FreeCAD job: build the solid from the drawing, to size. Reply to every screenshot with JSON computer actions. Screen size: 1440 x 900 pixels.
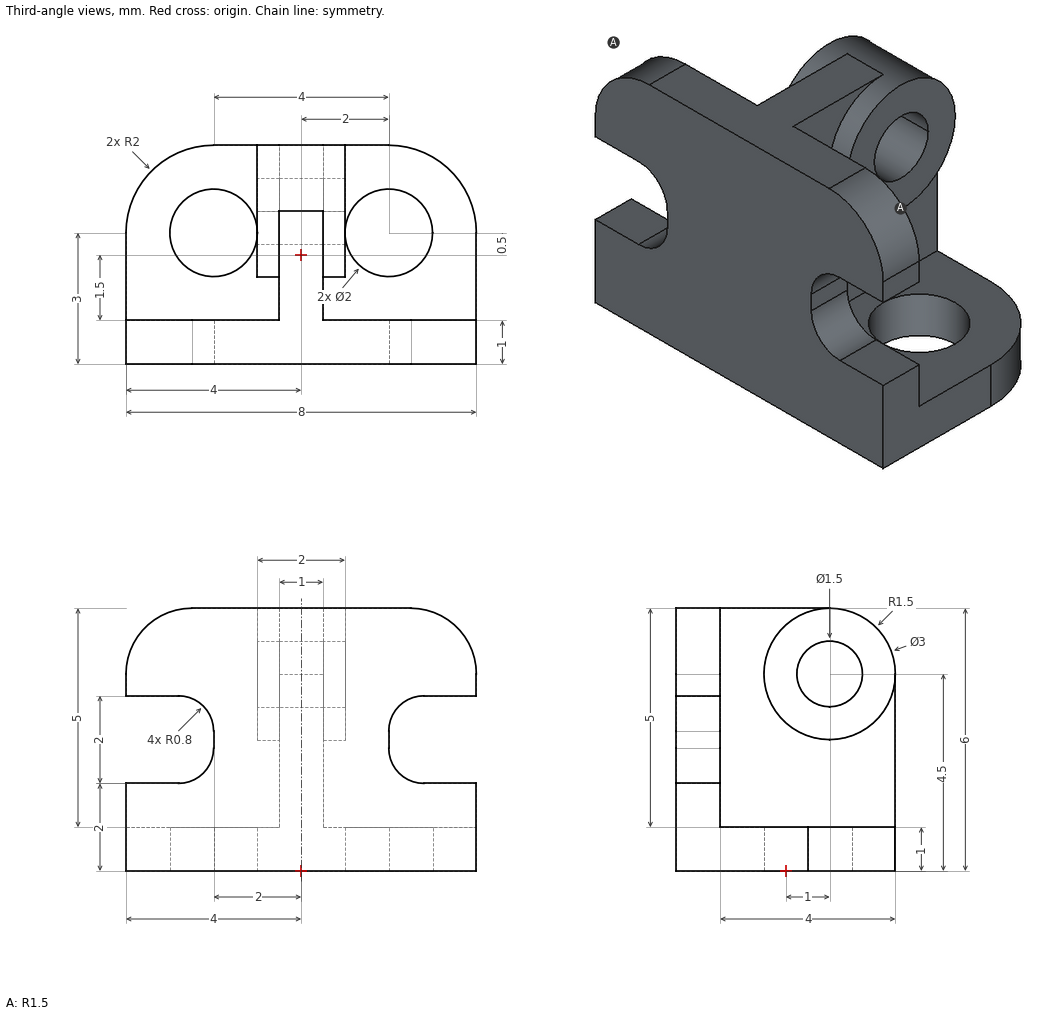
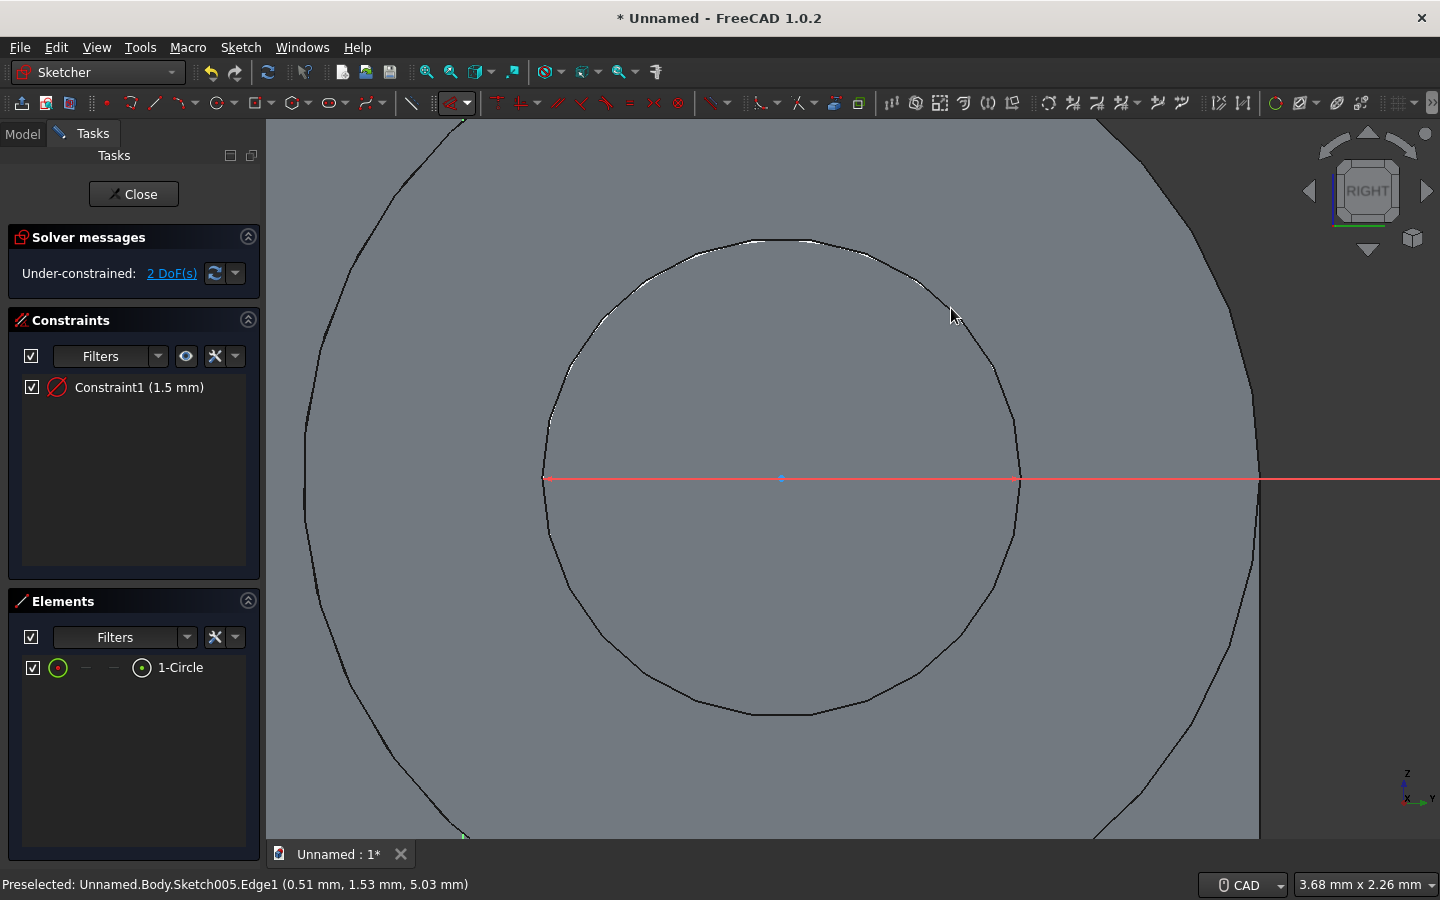
{"action": "left_click", "coordinate": [782, 479]}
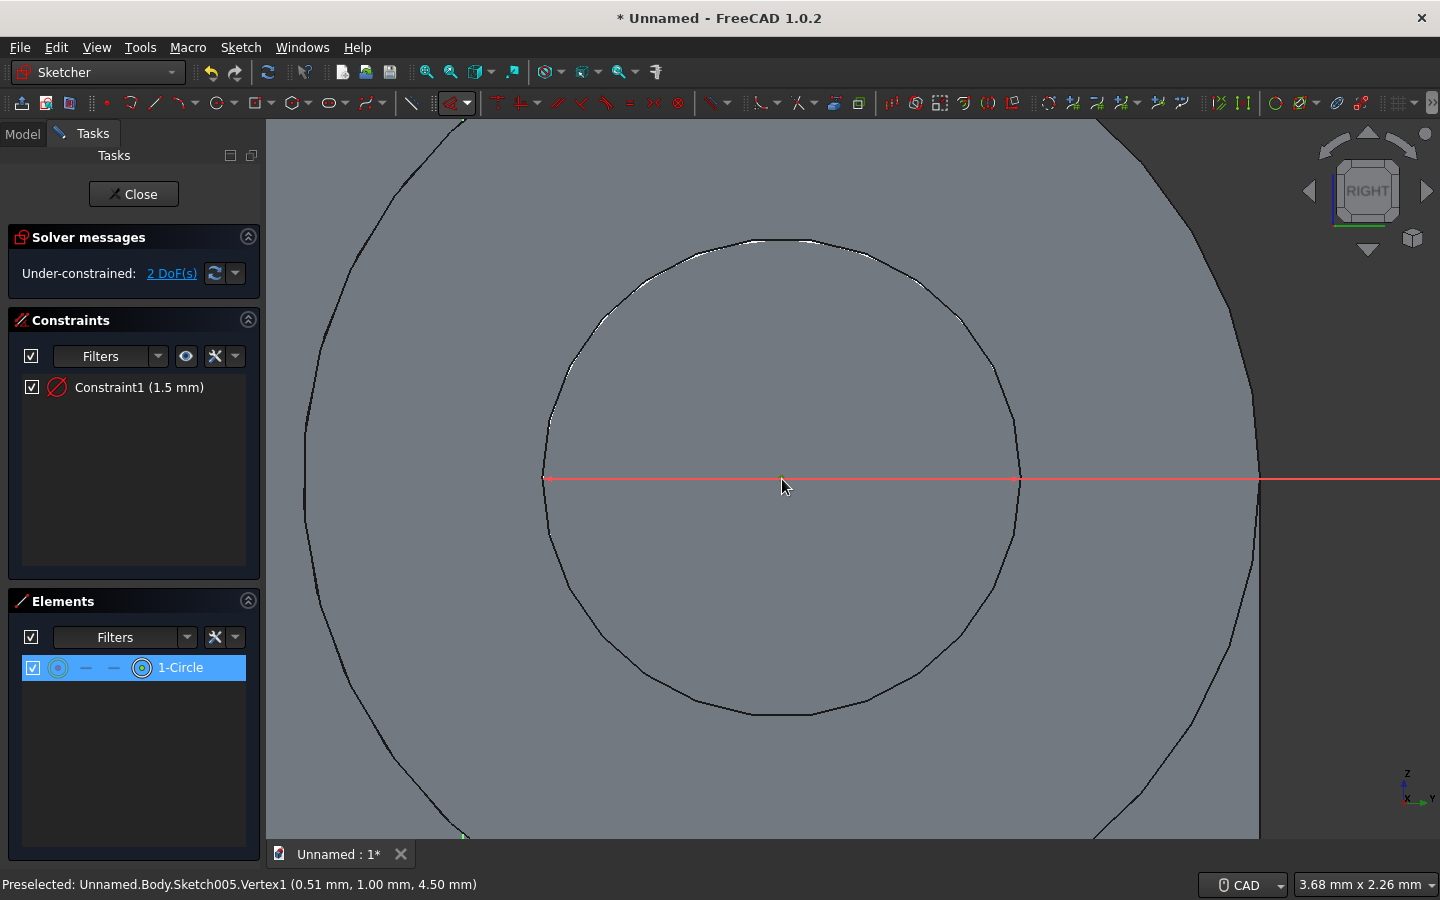
{"action": "left_click", "coordinate": [470, 104]}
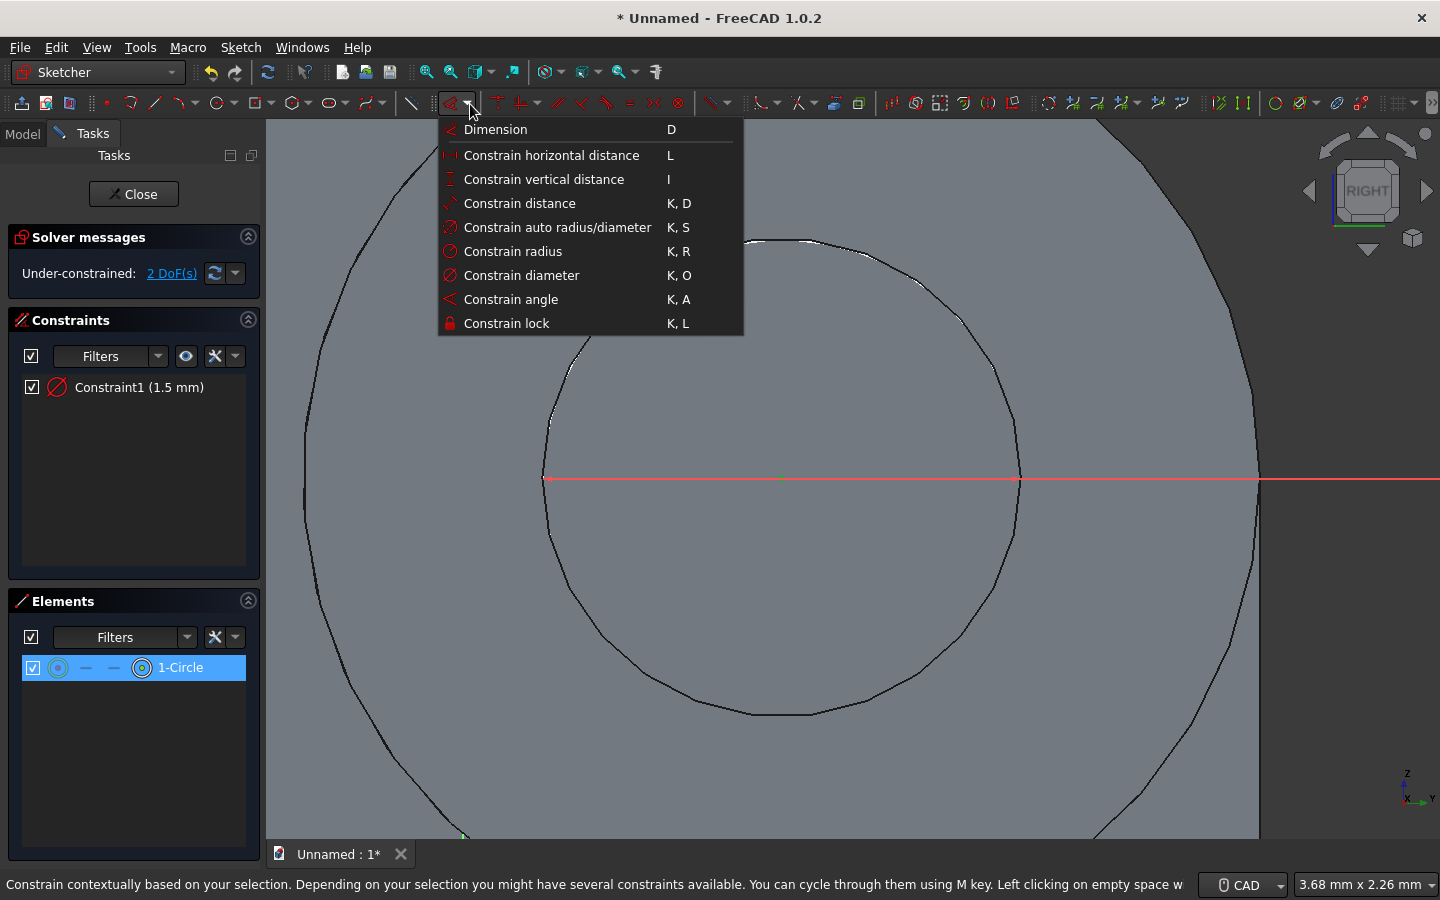
{"action": "left_click", "coordinate": [591, 155]}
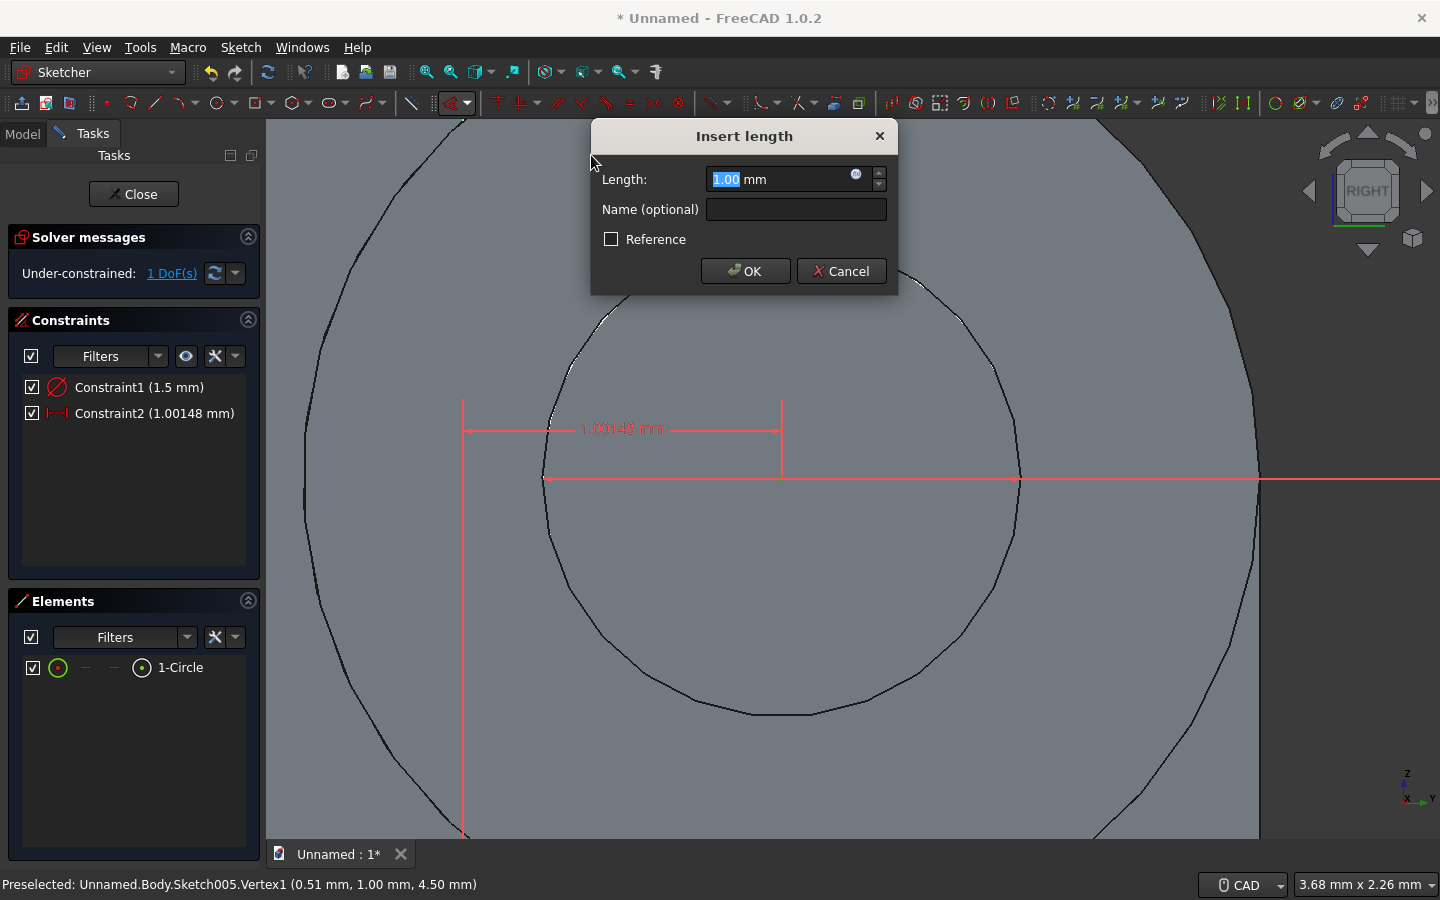
{"action": "type", "text": "1"}
{"action": "key", "text": "Return"}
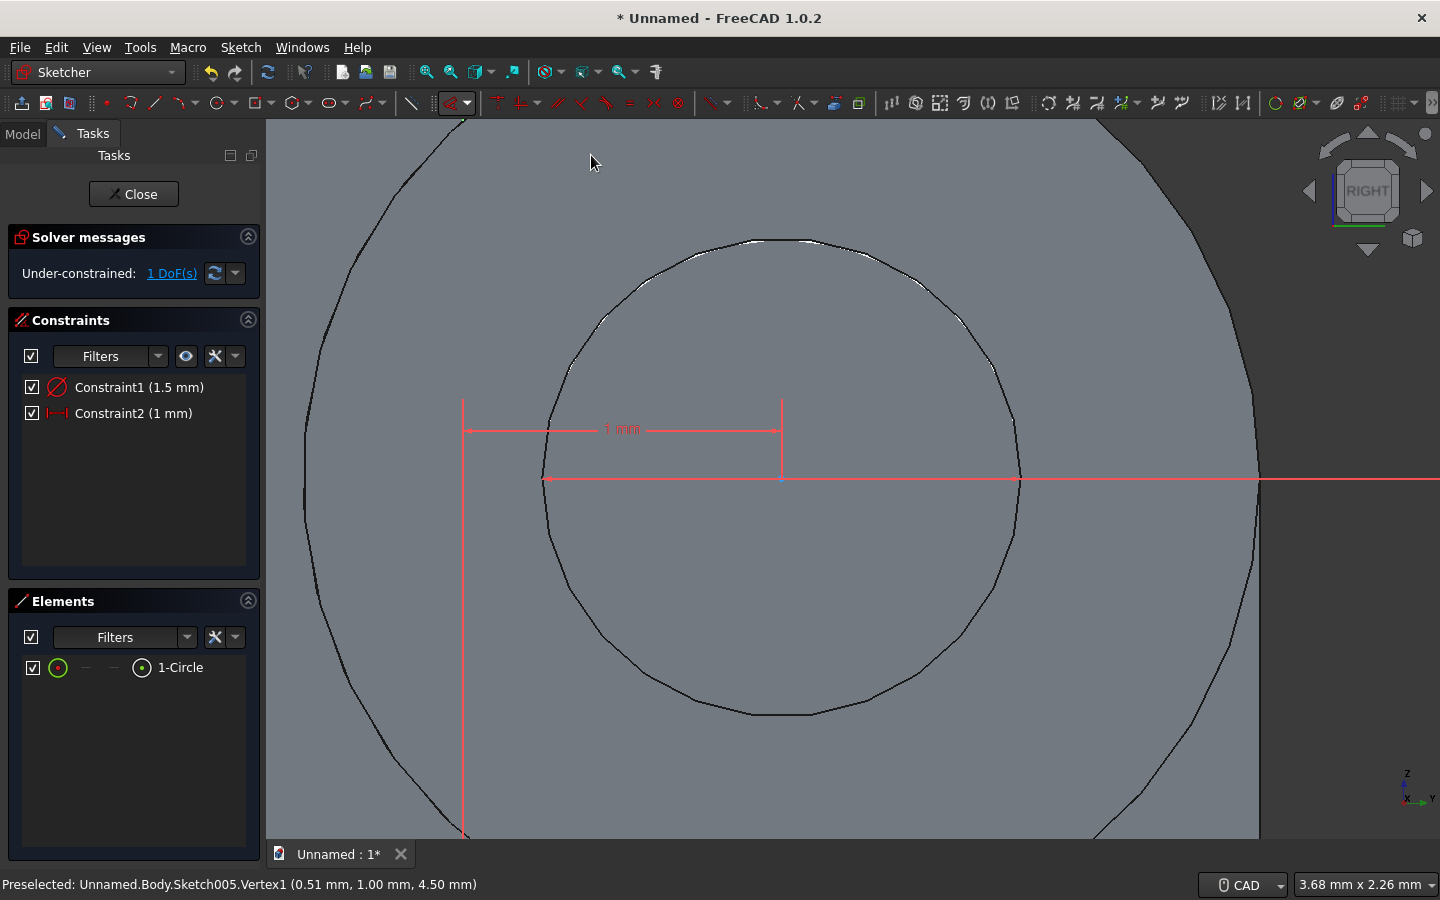
{"action": "left_click", "coordinate": [782, 479]}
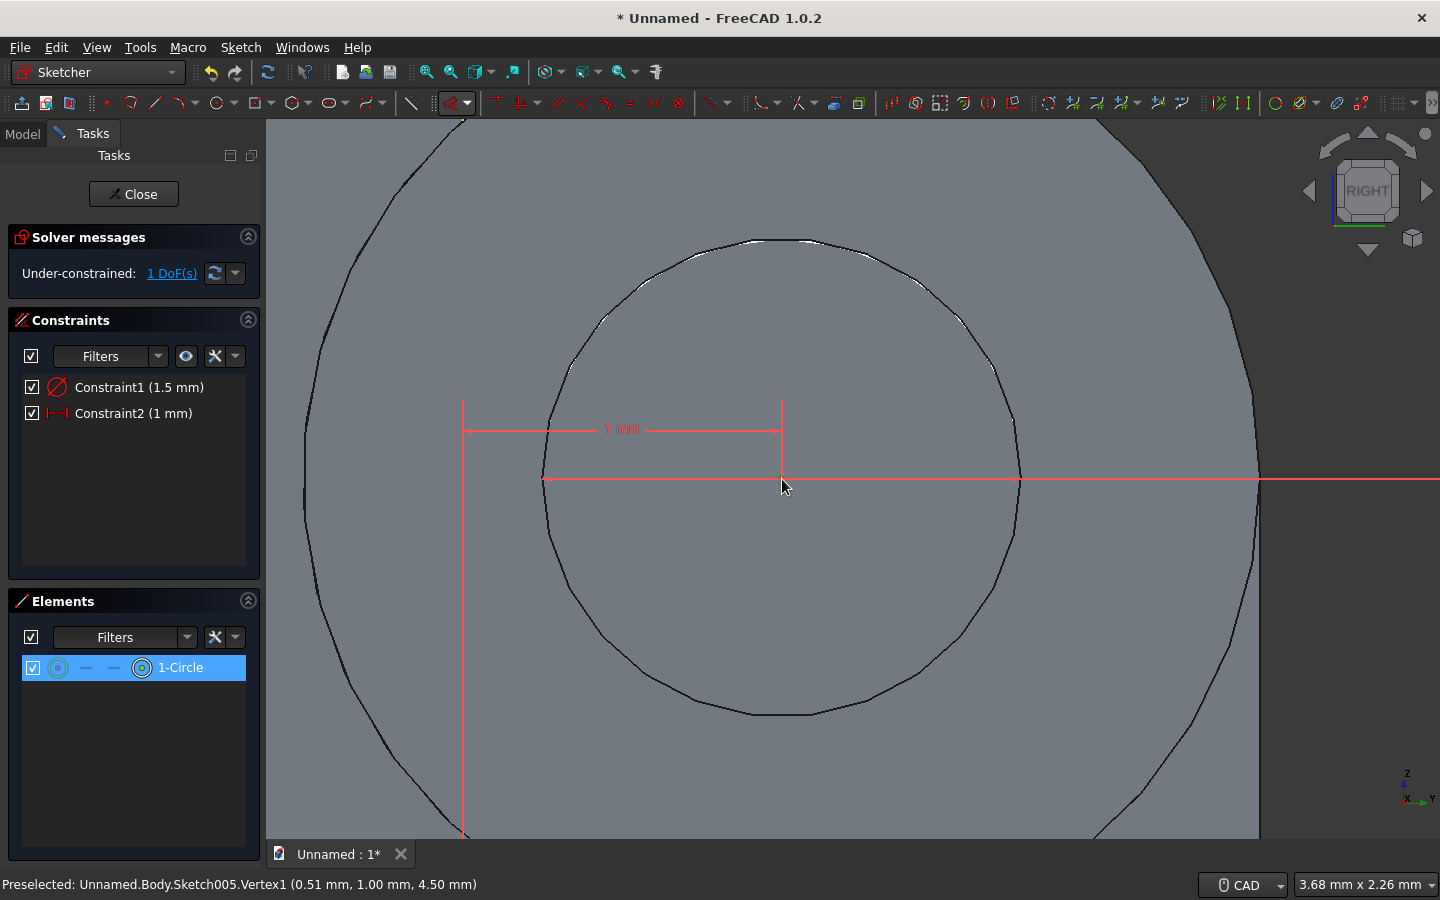
{"action": "left_click", "coordinate": [470, 104]}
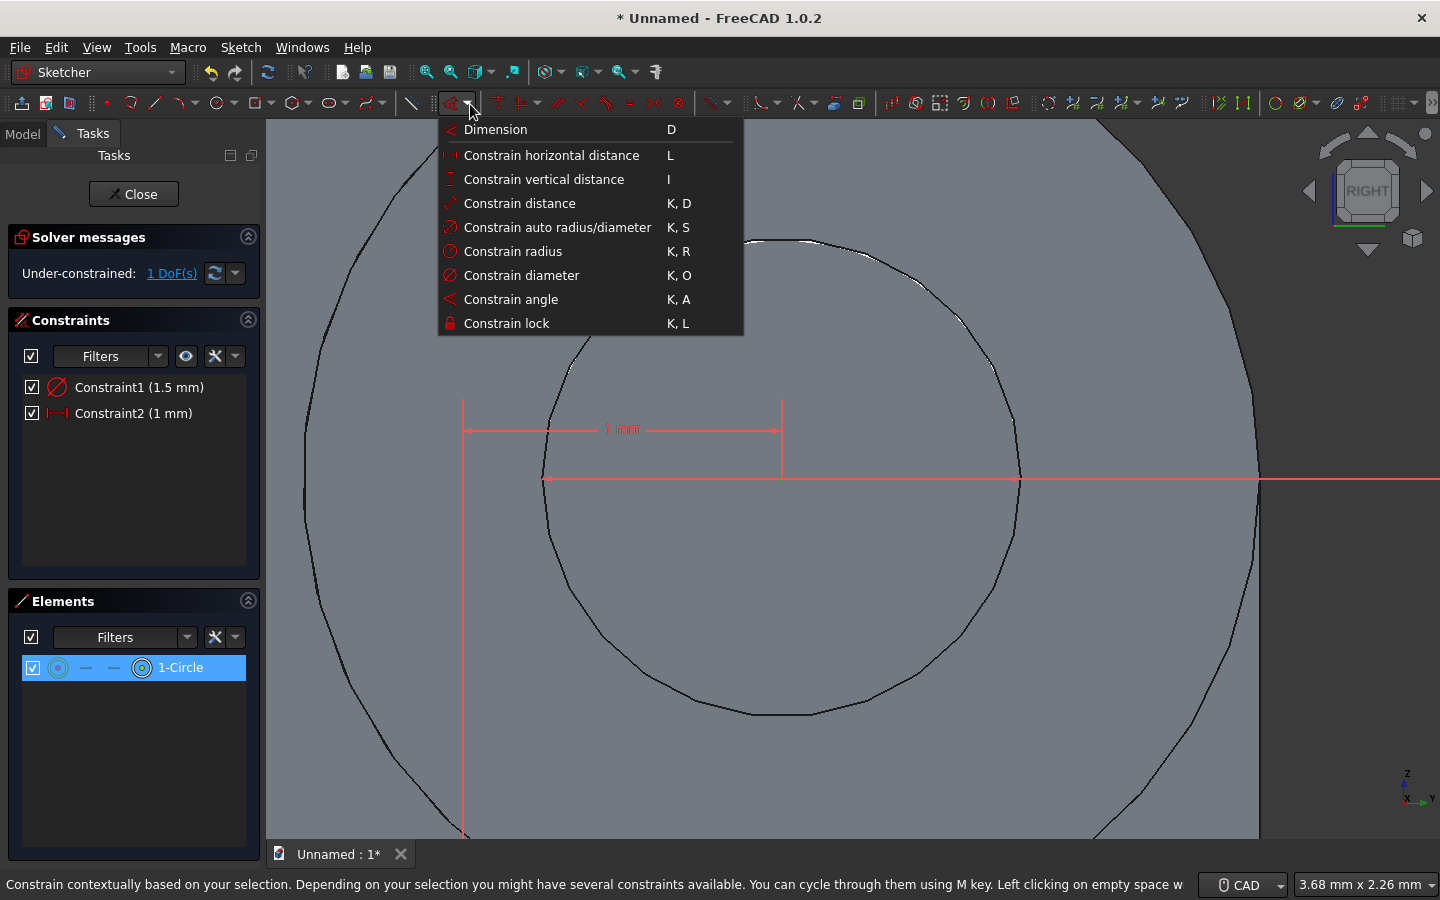
{"action": "left_click", "coordinate": [591, 179]}